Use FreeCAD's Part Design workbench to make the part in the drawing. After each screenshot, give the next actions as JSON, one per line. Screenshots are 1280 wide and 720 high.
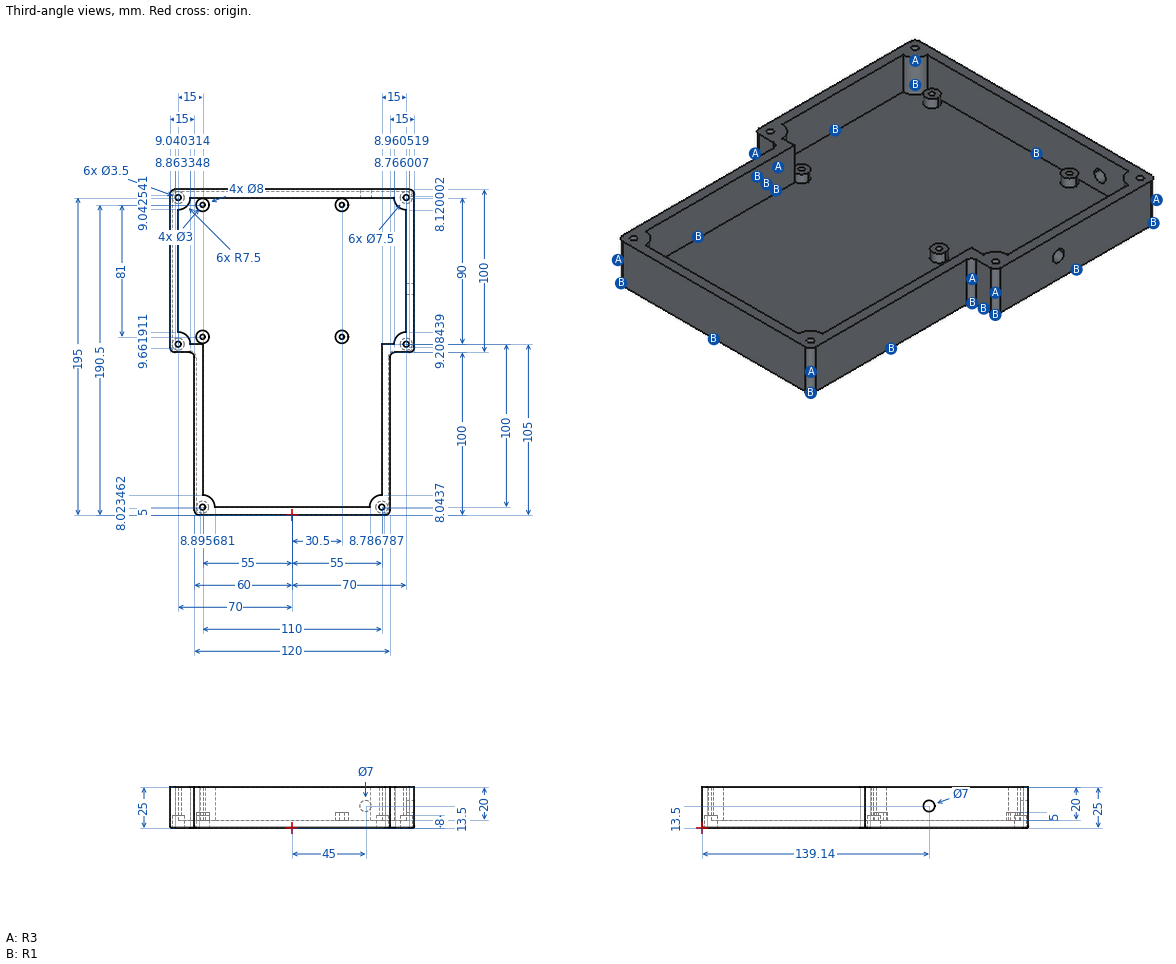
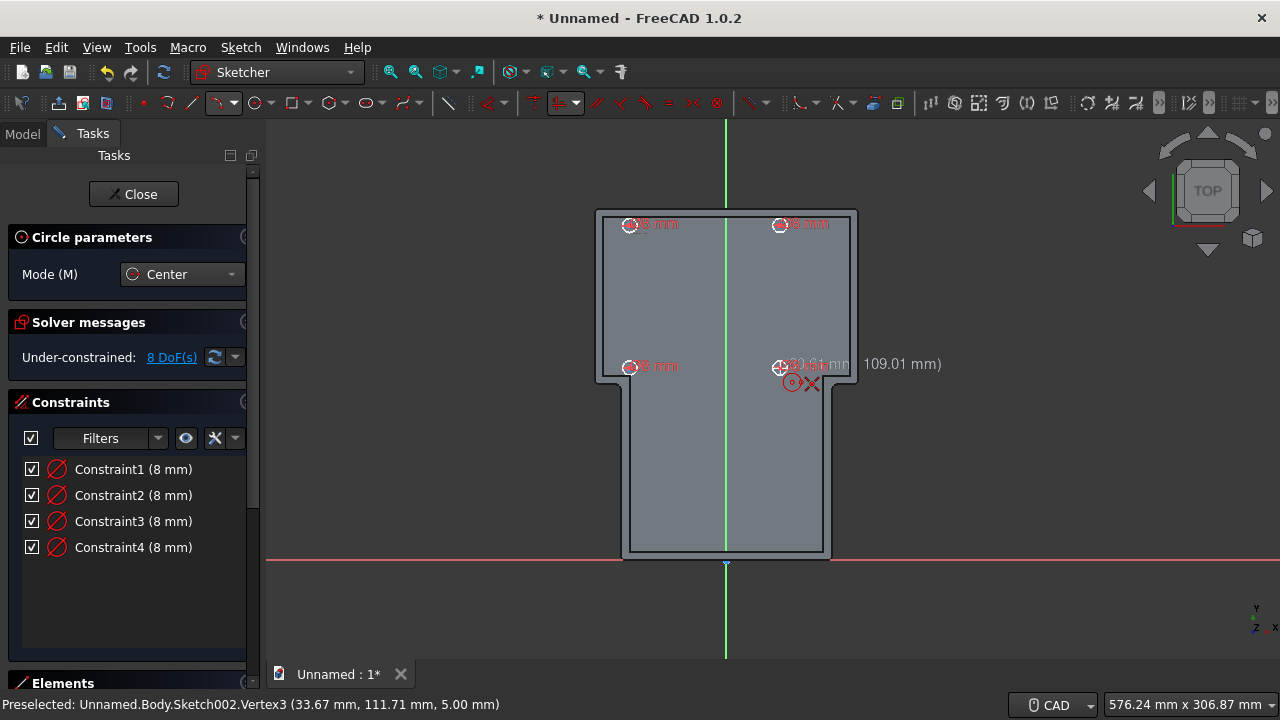
{"action": "scroll", "coordinate": [630, 225], "scroll_direction": "up", "scroll_amount": 11}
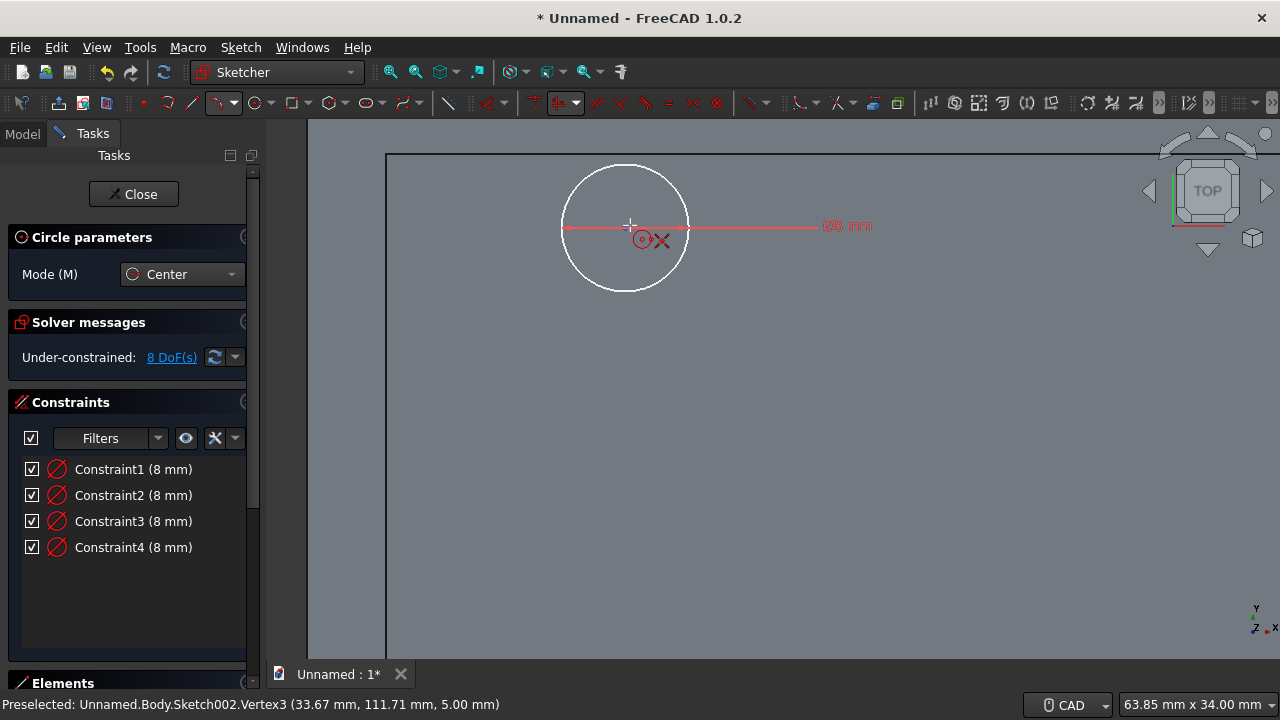
{"action": "scroll", "coordinate": [630, 225], "scroll_direction": "down", "scroll_amount": 11}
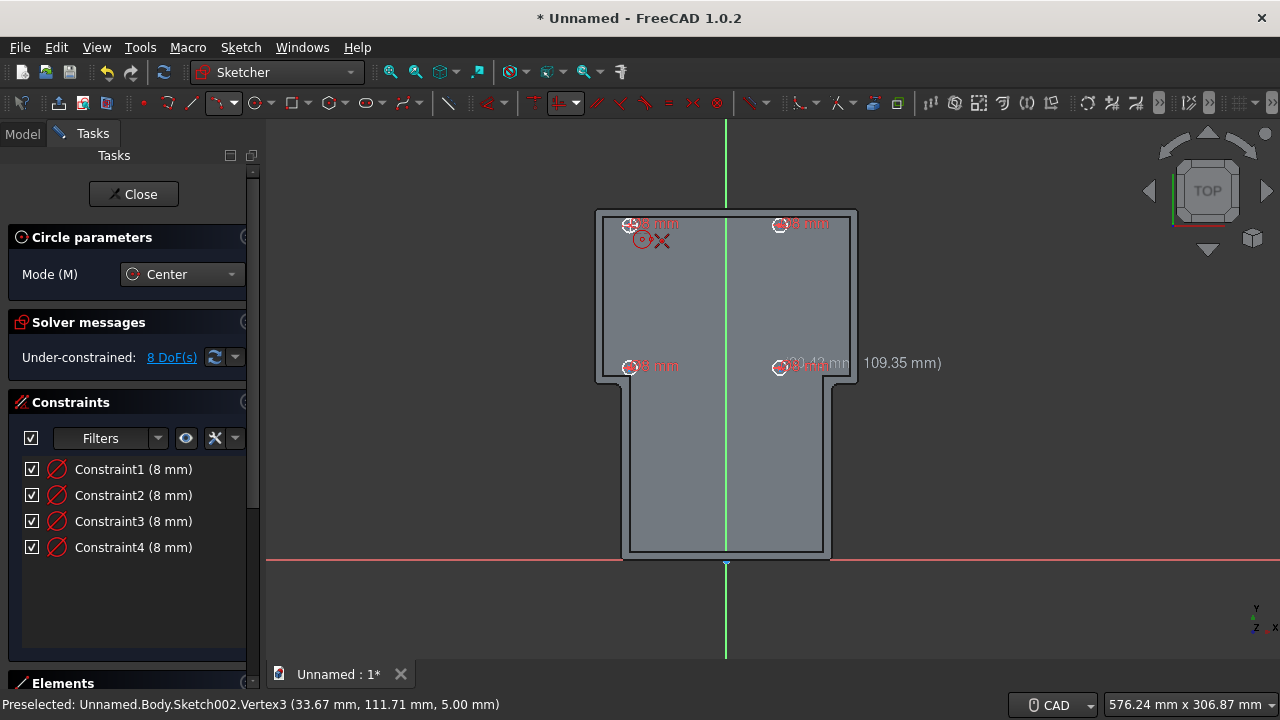
{"action": "scroll", "coordinate": [630, 225], "scroll_direction": "up", "scroll_amount": 5}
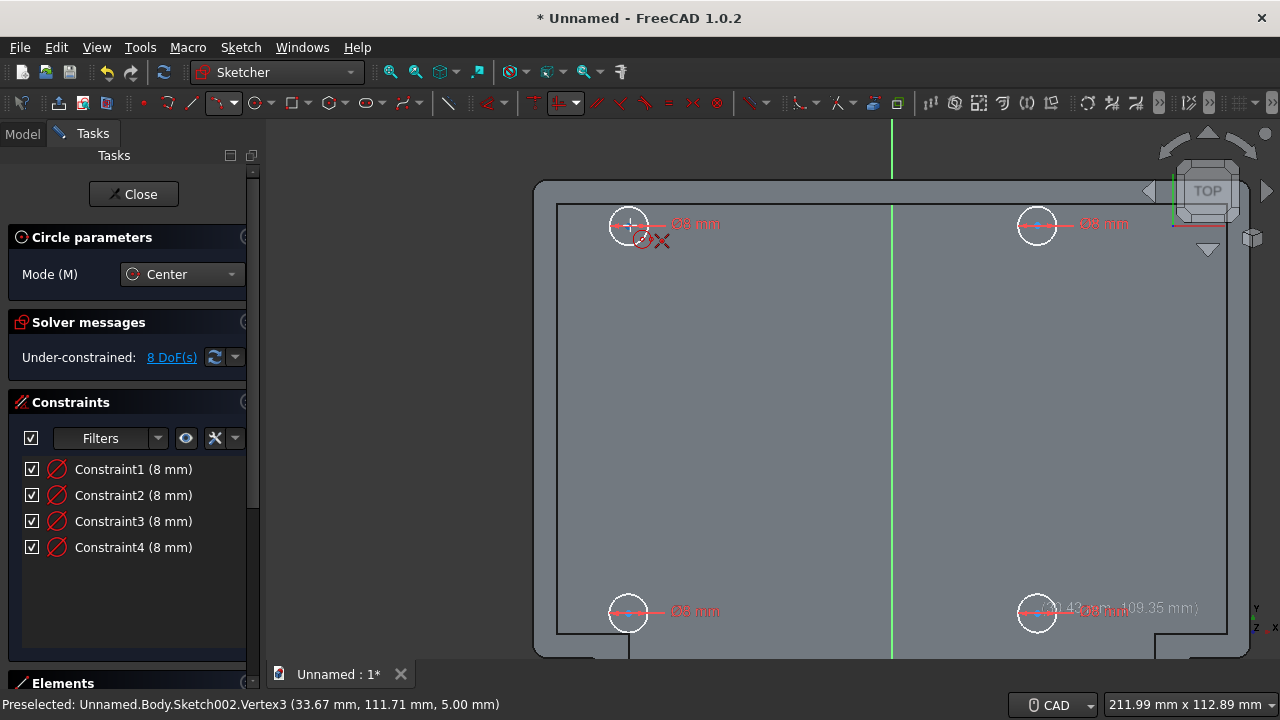
{"action": "left_click", "coordinate": [629, 226]}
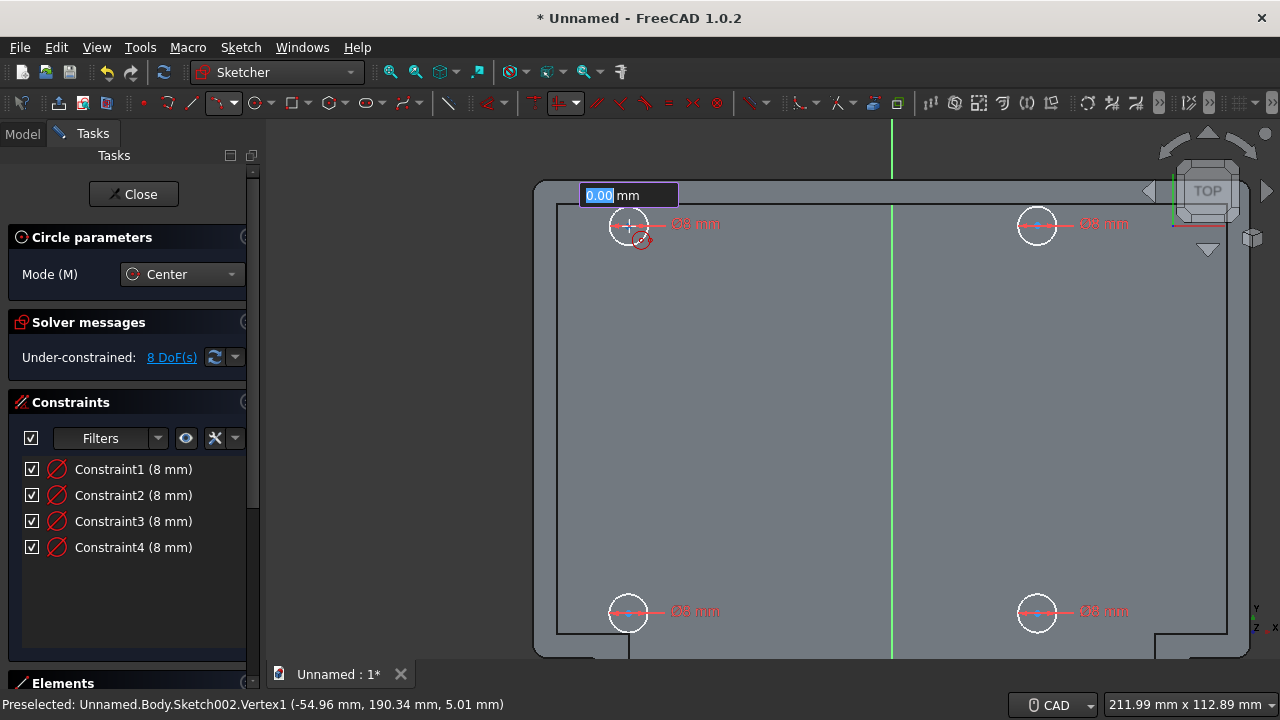
{"action": "scroll", "coordinate": [631, 219], "scroll_direction": "up", "scroll_amount": 4}
{"action": "mouse_move", "coordinate": [631, 218]}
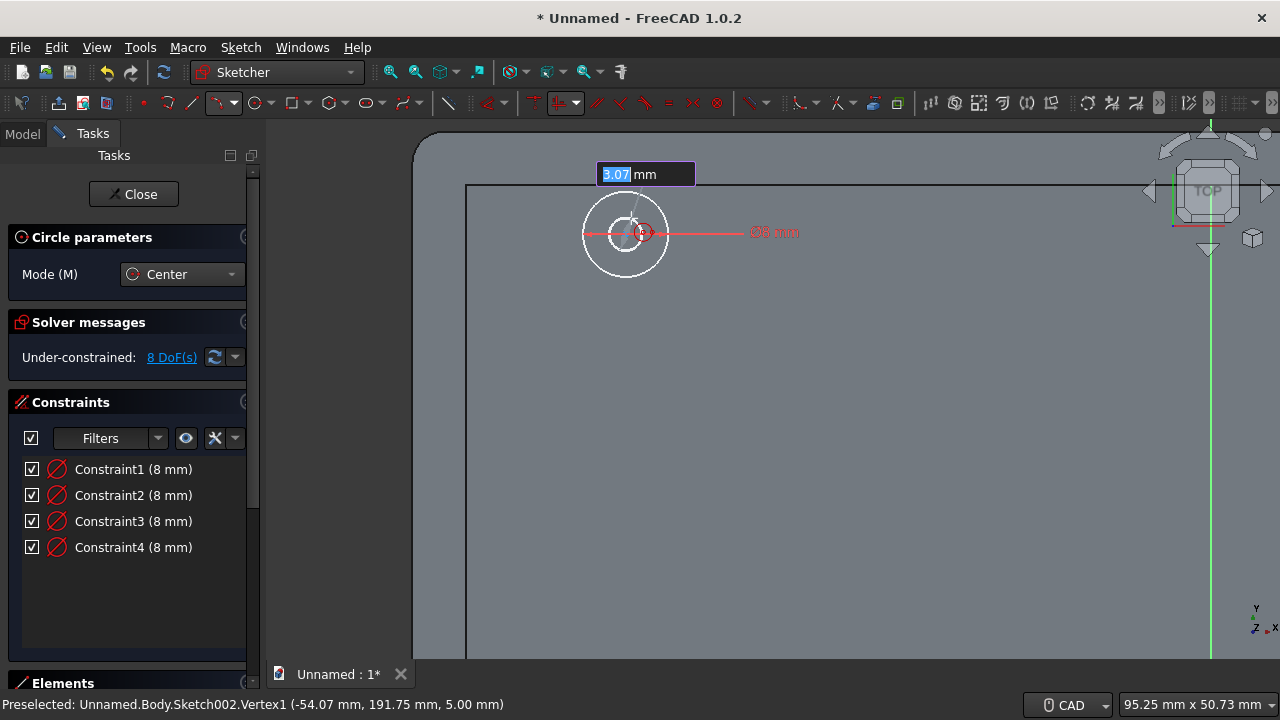
{"action": "type", "text": "3"}
{"action": "key", "text": "Return"}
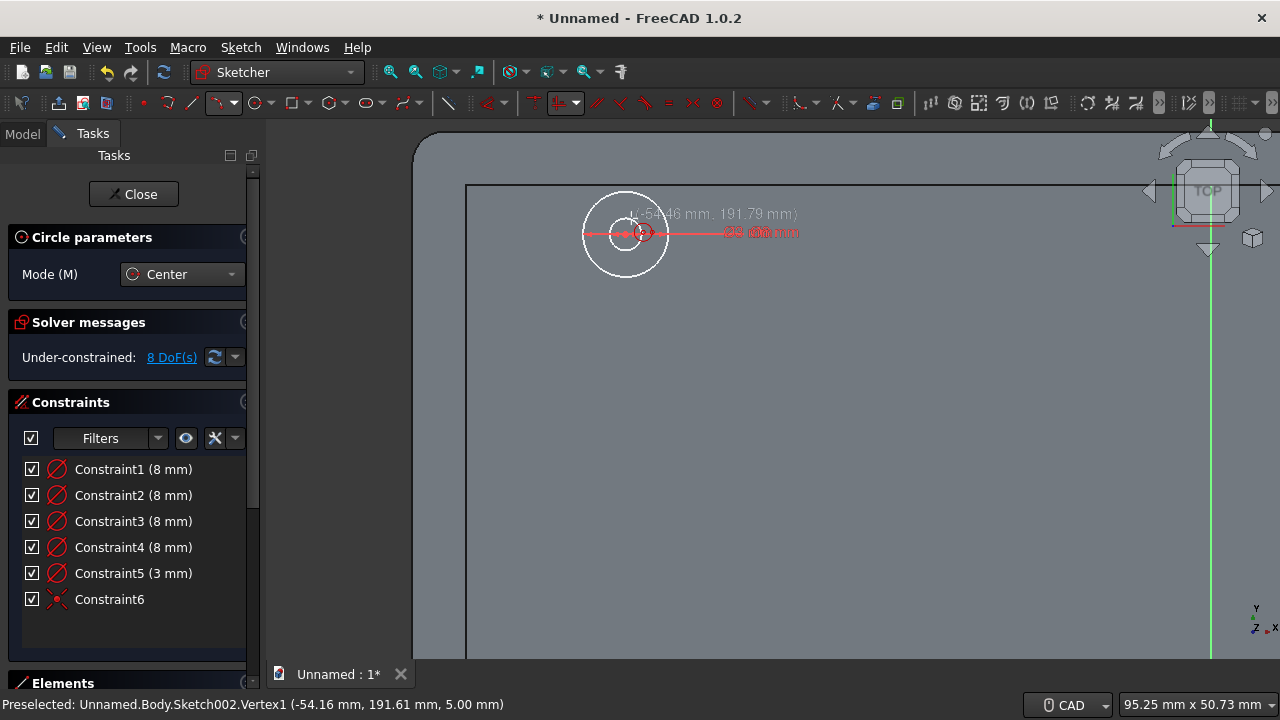
{"action": "scroll", "coordinate": [630, 223], "scroll_direction": "down", "scroll_amount": 9}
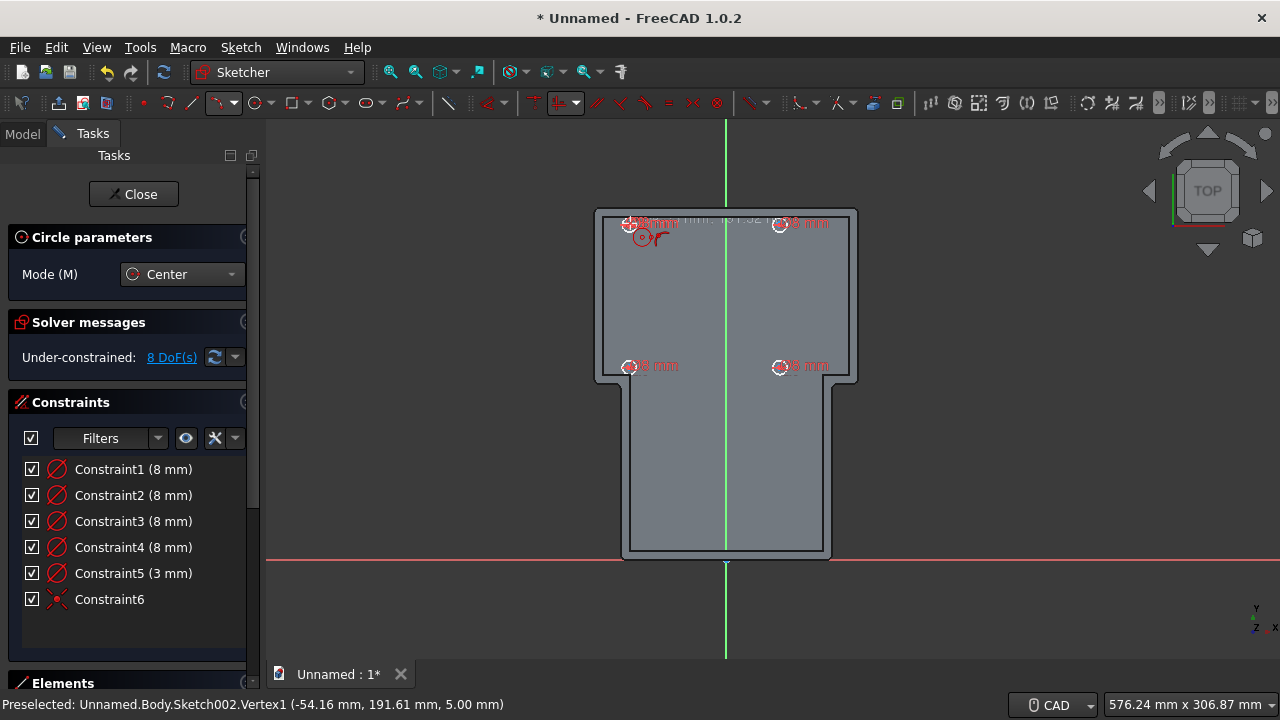
{"action": "scroll", "coordinate": [780, 225], "scroll_direction": "up", "scroll_amount": 11}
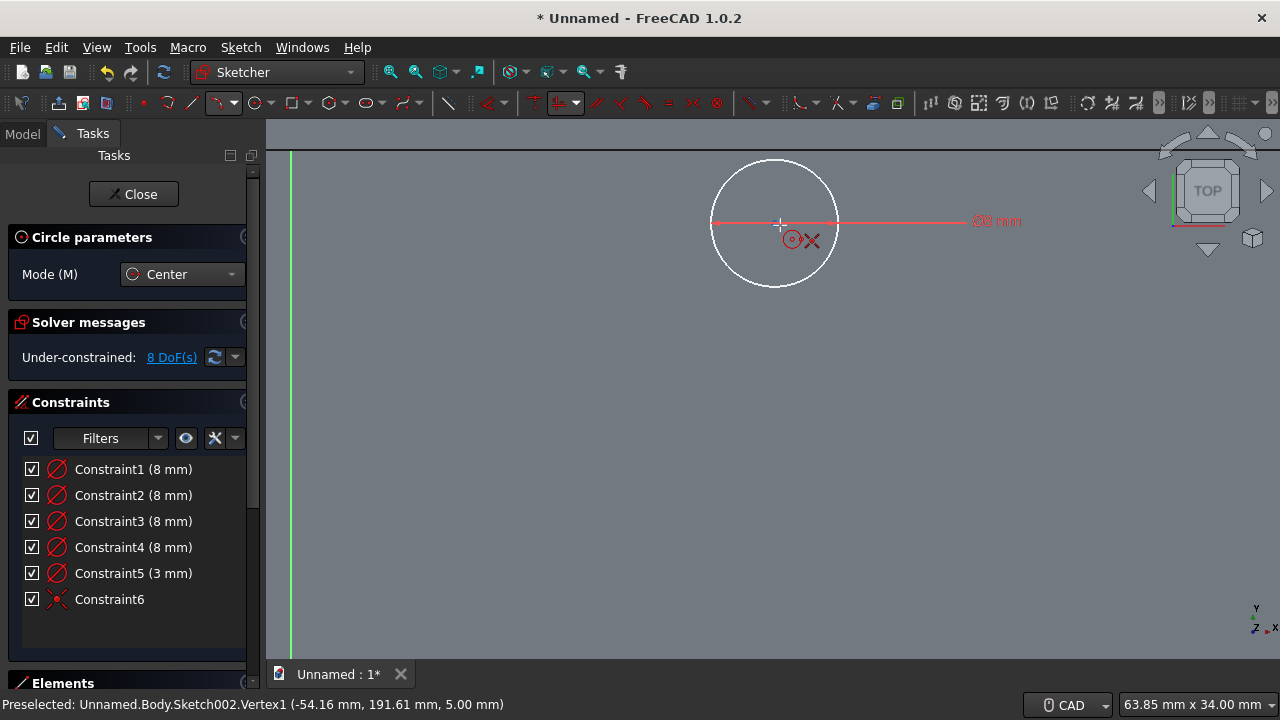
{"action": "scroll", "coordinate": [780, 225], "scroll_direction": "down", "scroll_amount": 11}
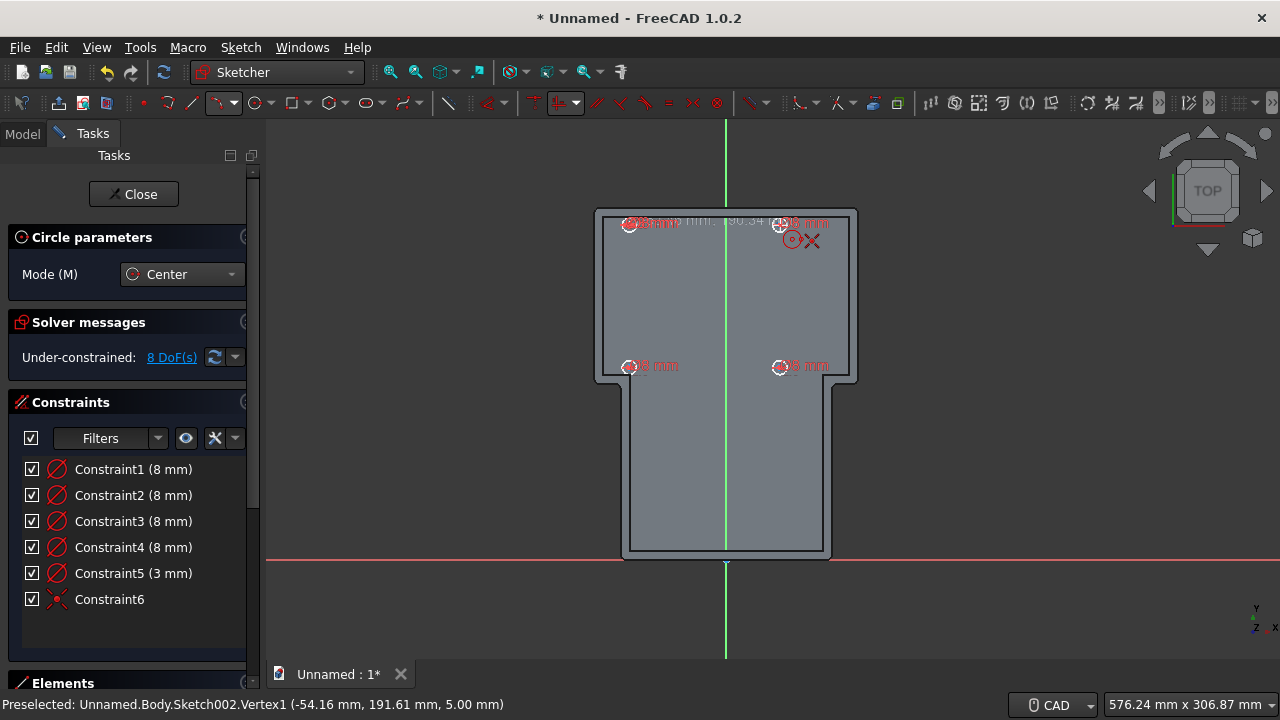
{"action": "scroll", "coordinate": [780, 225], "scroll_direction": "up", "scroll_amount": 5}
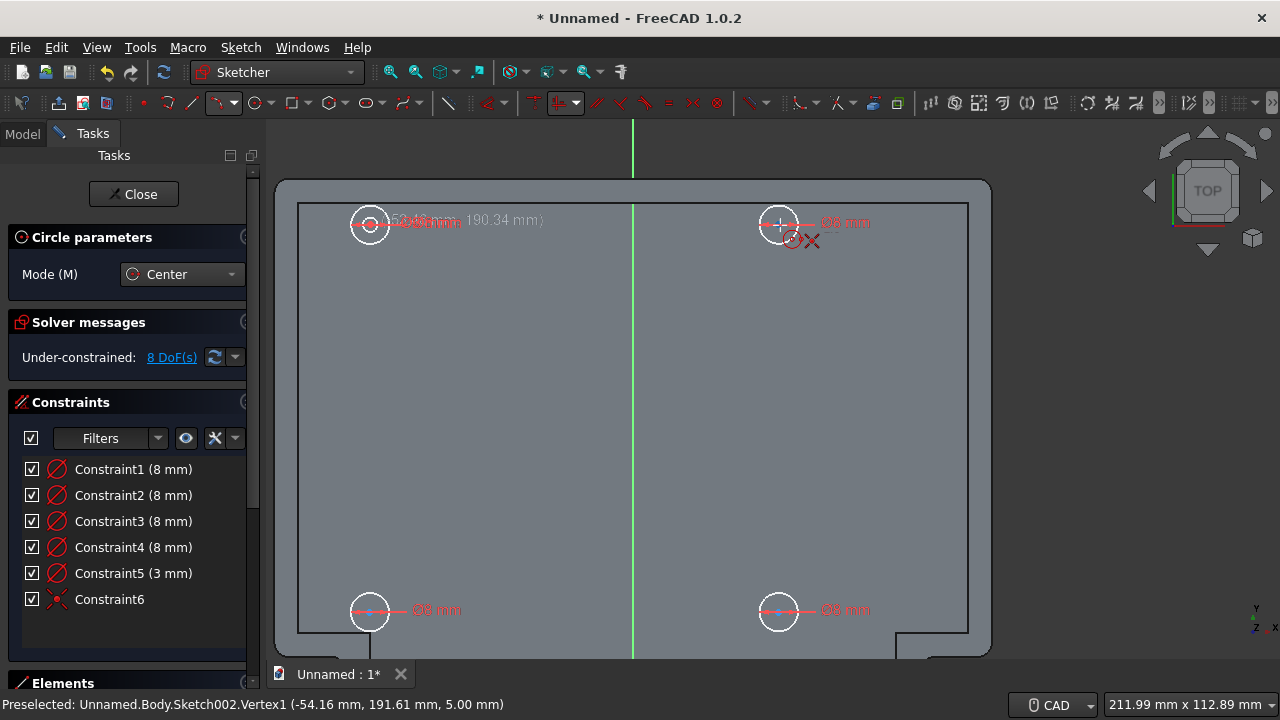
{"action": "left_click", "coordinate": [779, 225]}